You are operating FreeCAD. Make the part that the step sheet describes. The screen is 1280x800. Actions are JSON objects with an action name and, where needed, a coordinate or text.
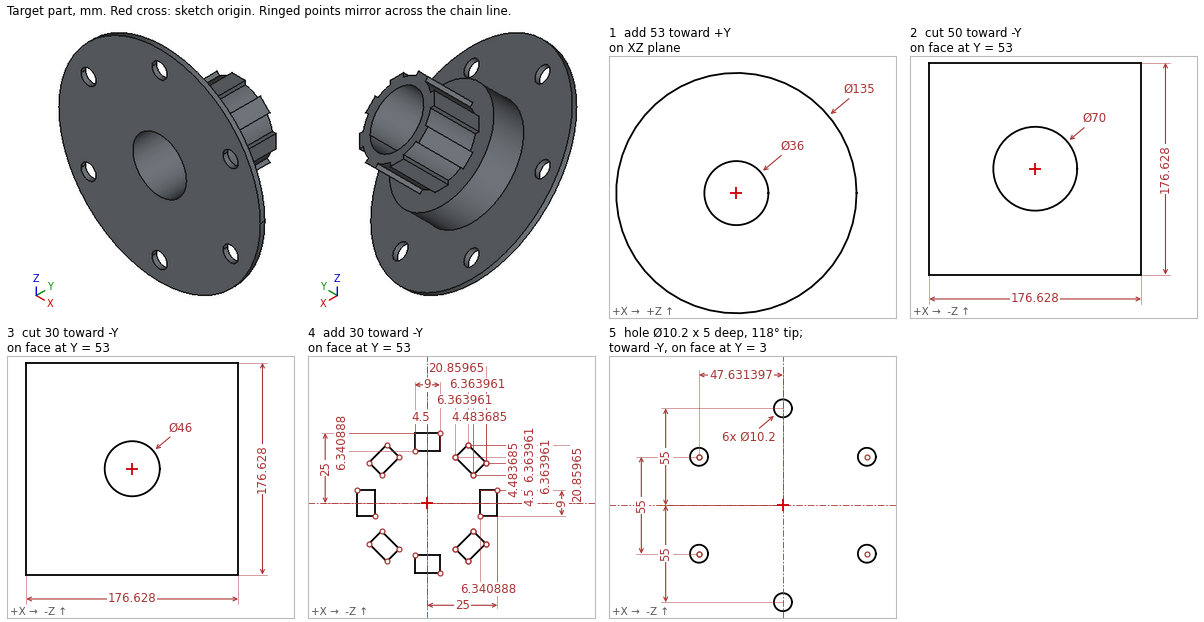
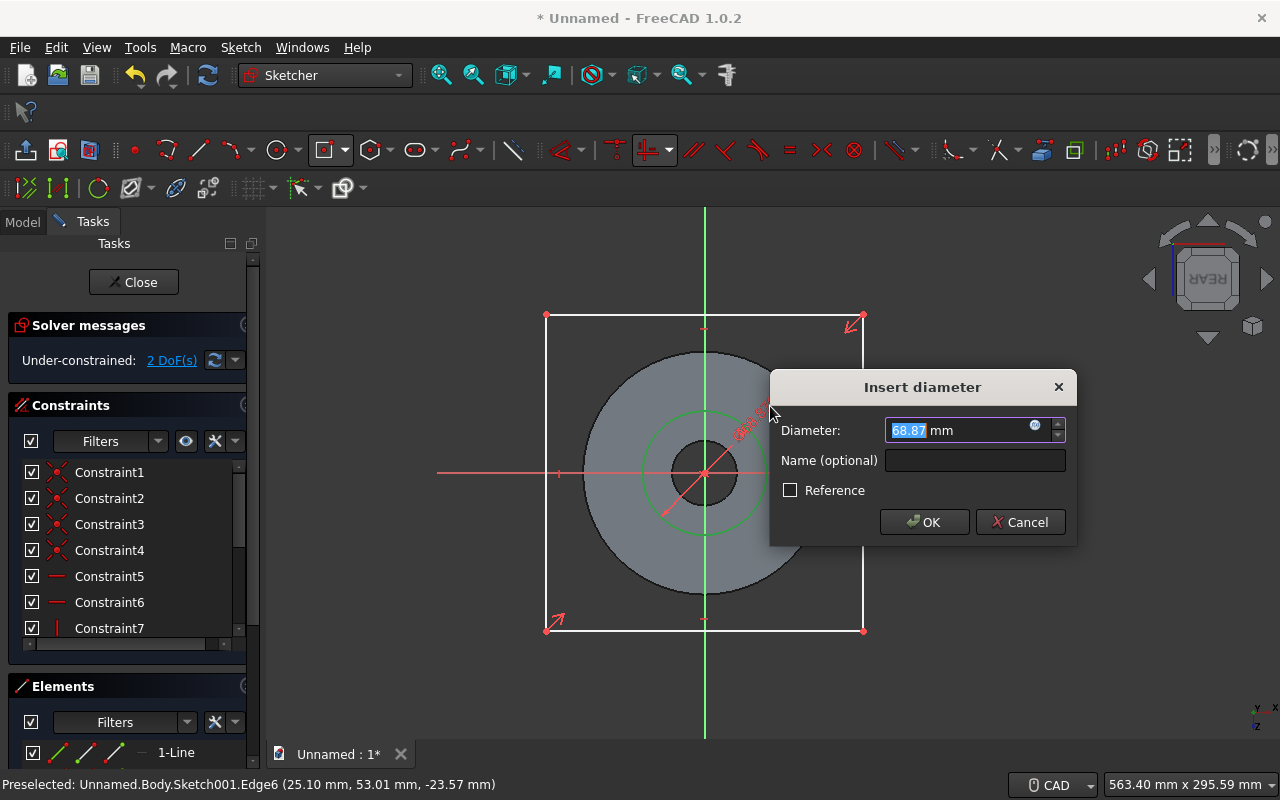
{"action": "type", "text": "70"}
{"action": "key", "text": "Return"}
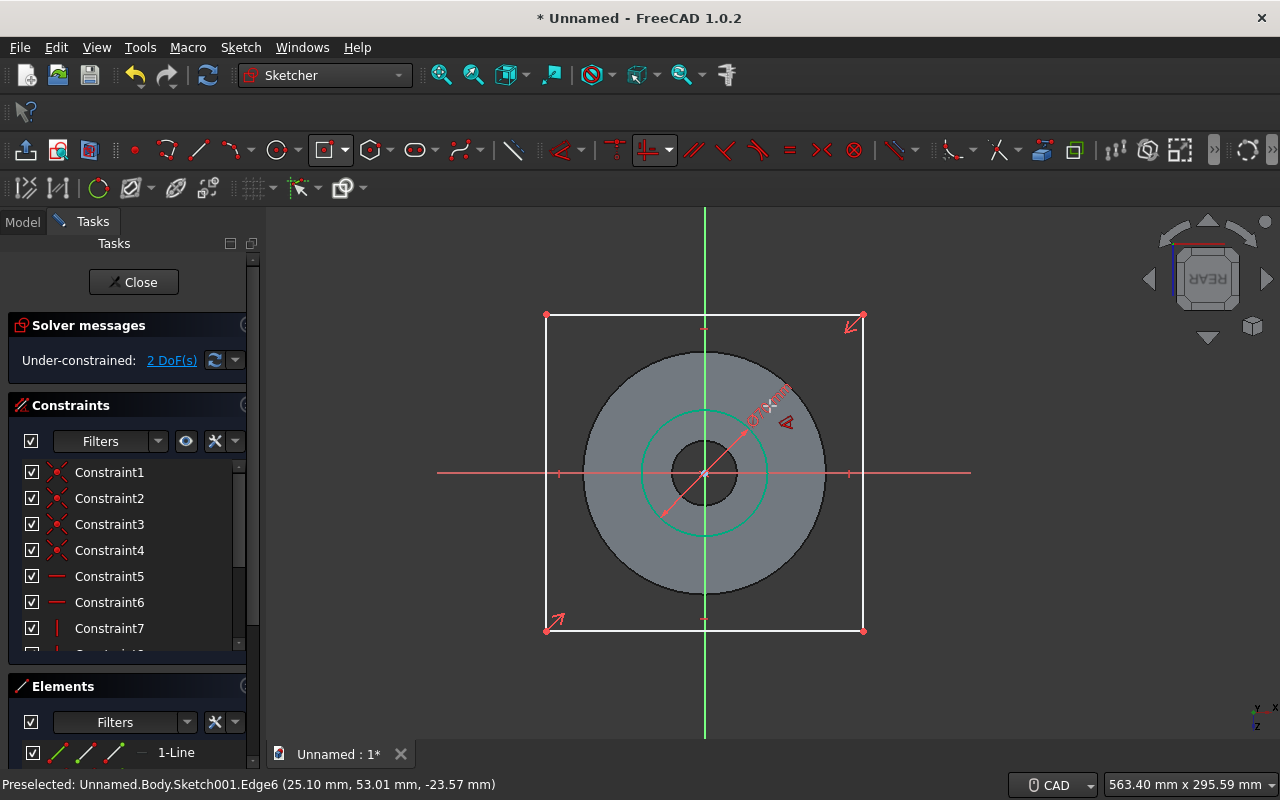
{"action": "left_click", "coordinate": [641, 631]}
{"action": "left_click", "coordinate": [632, 665]}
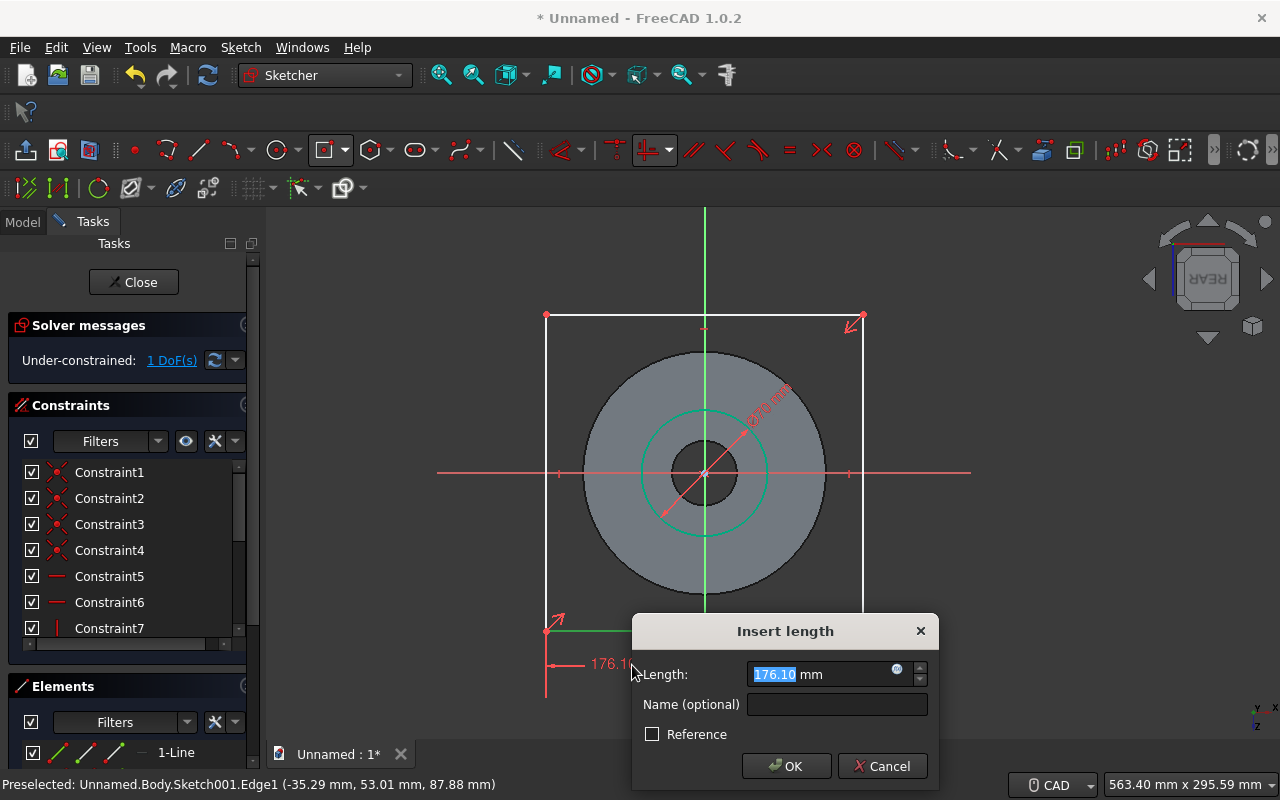
{"action": "type", "text": "176.628"}
{"action": "key", "text": "Return"}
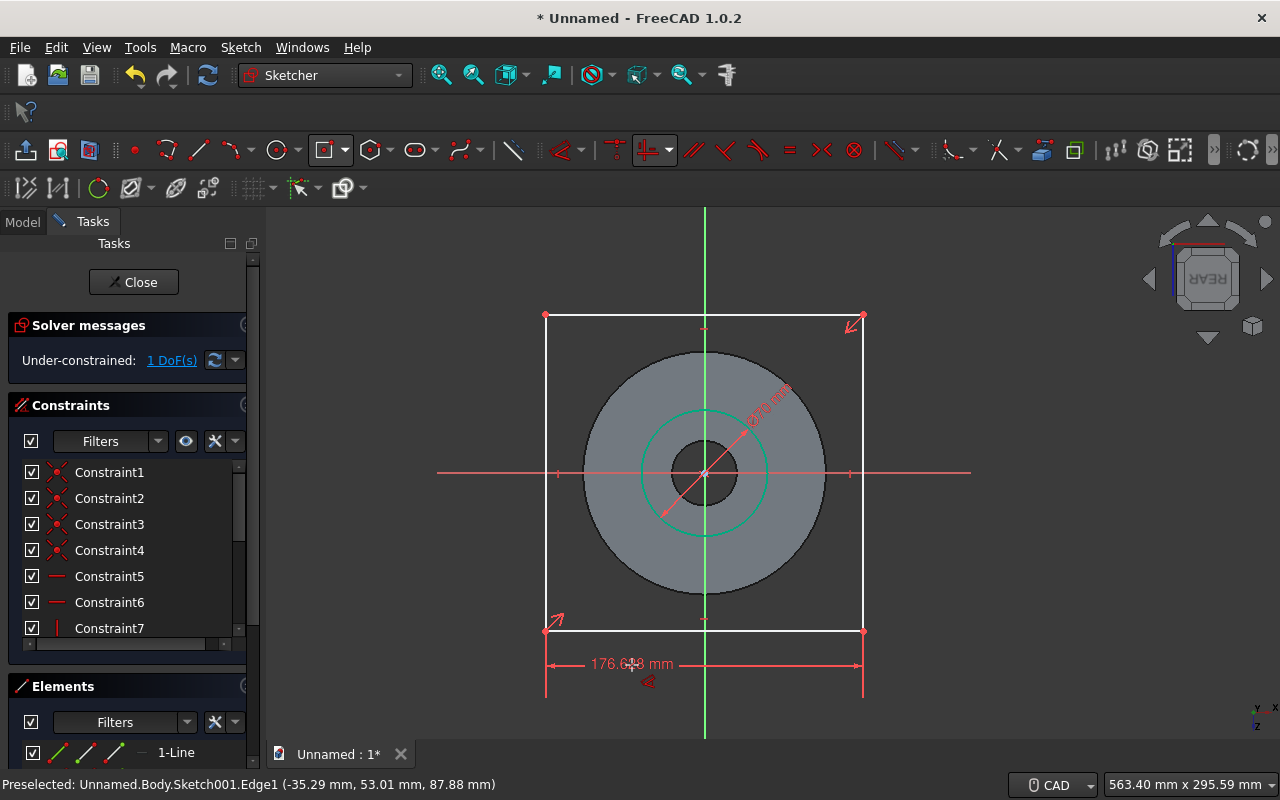
{"action": "left_click", "coordinate": [863, 536]}
{"action": "left_click", "coordinate": [897, 400]}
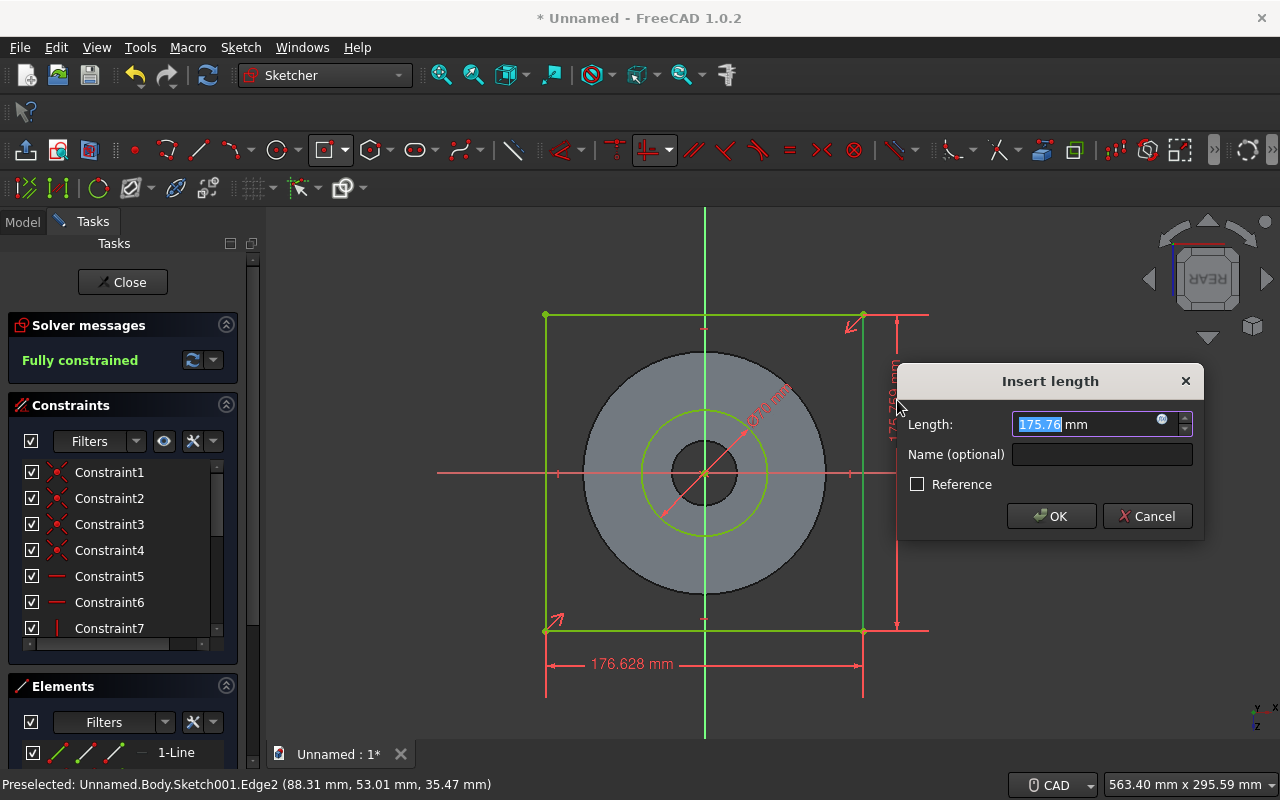
{"action": "type", "text": "176.628"}
{"action": "key", "text": "Return"}
{"action": "key", "text": "Escape"}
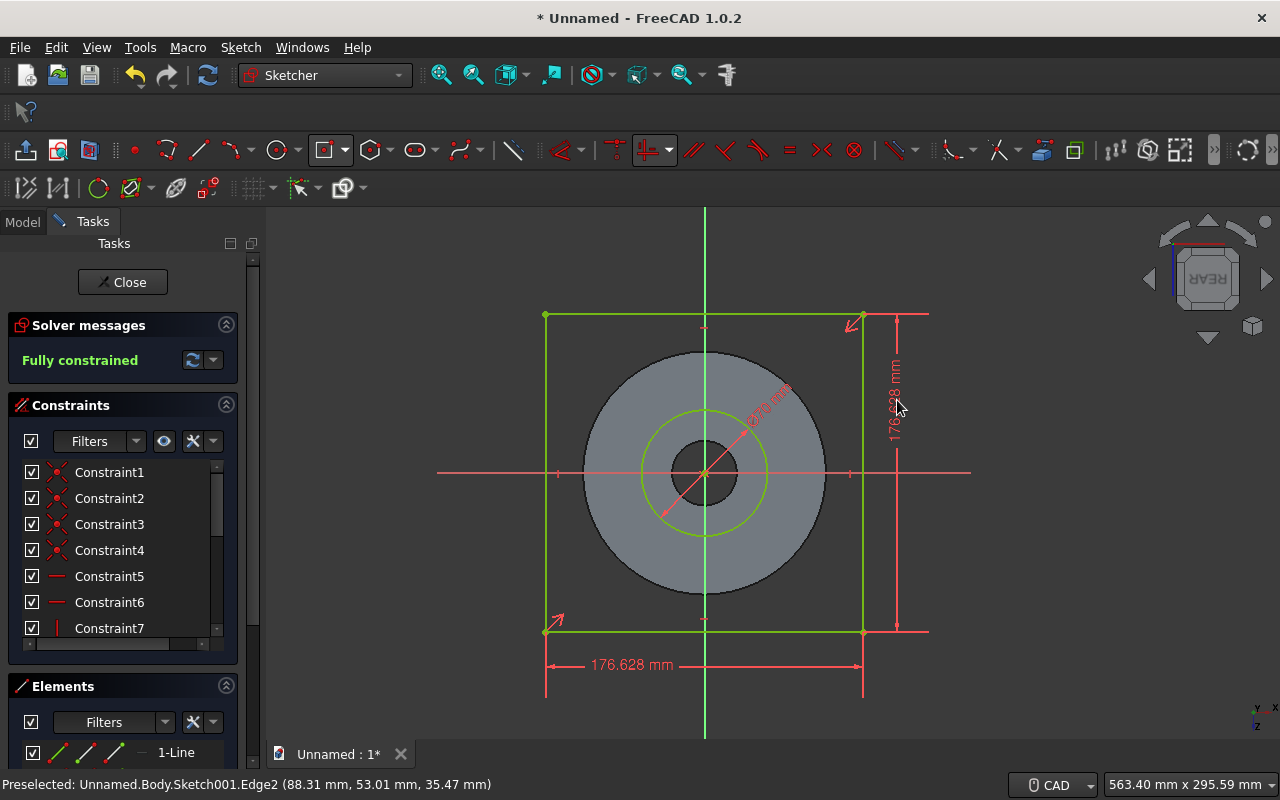
{"action": "left_click", "coordinate": [123, 282]}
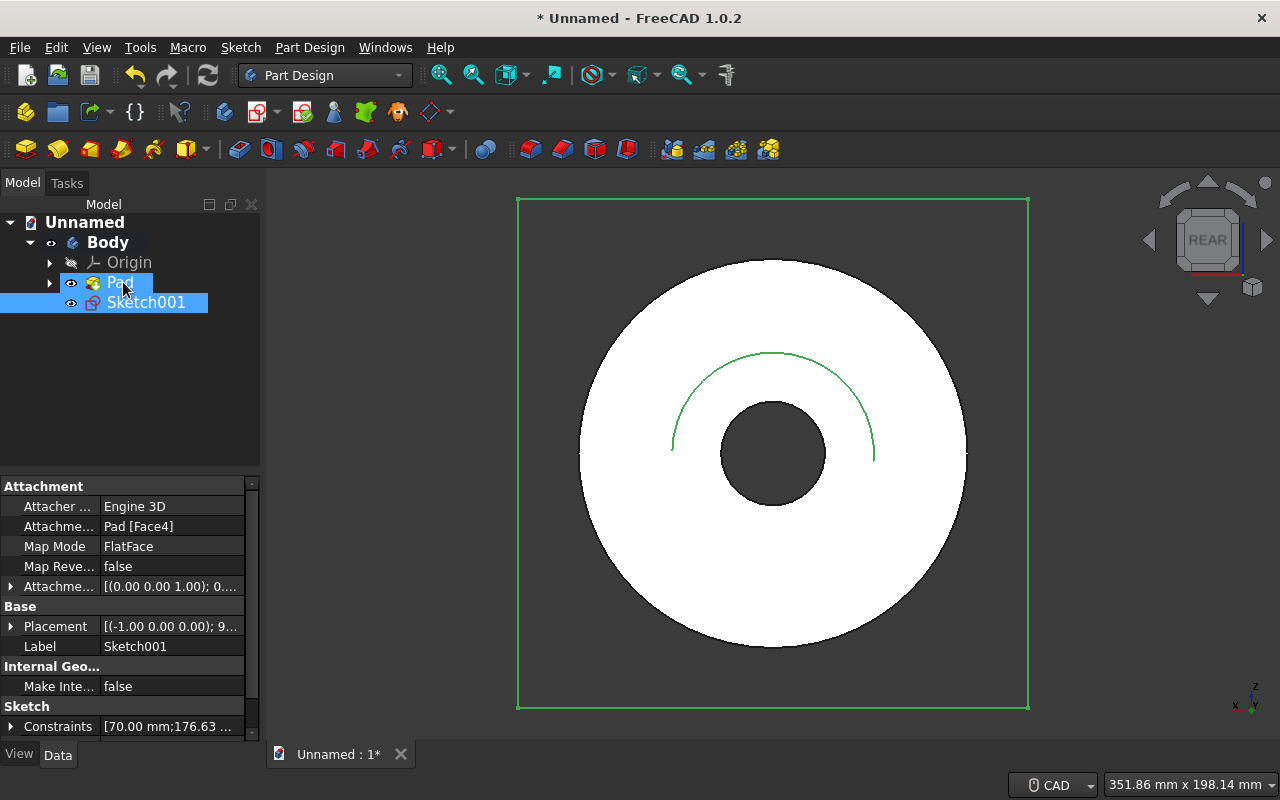
{"action": "left_click", "coordinate": [240, 150]}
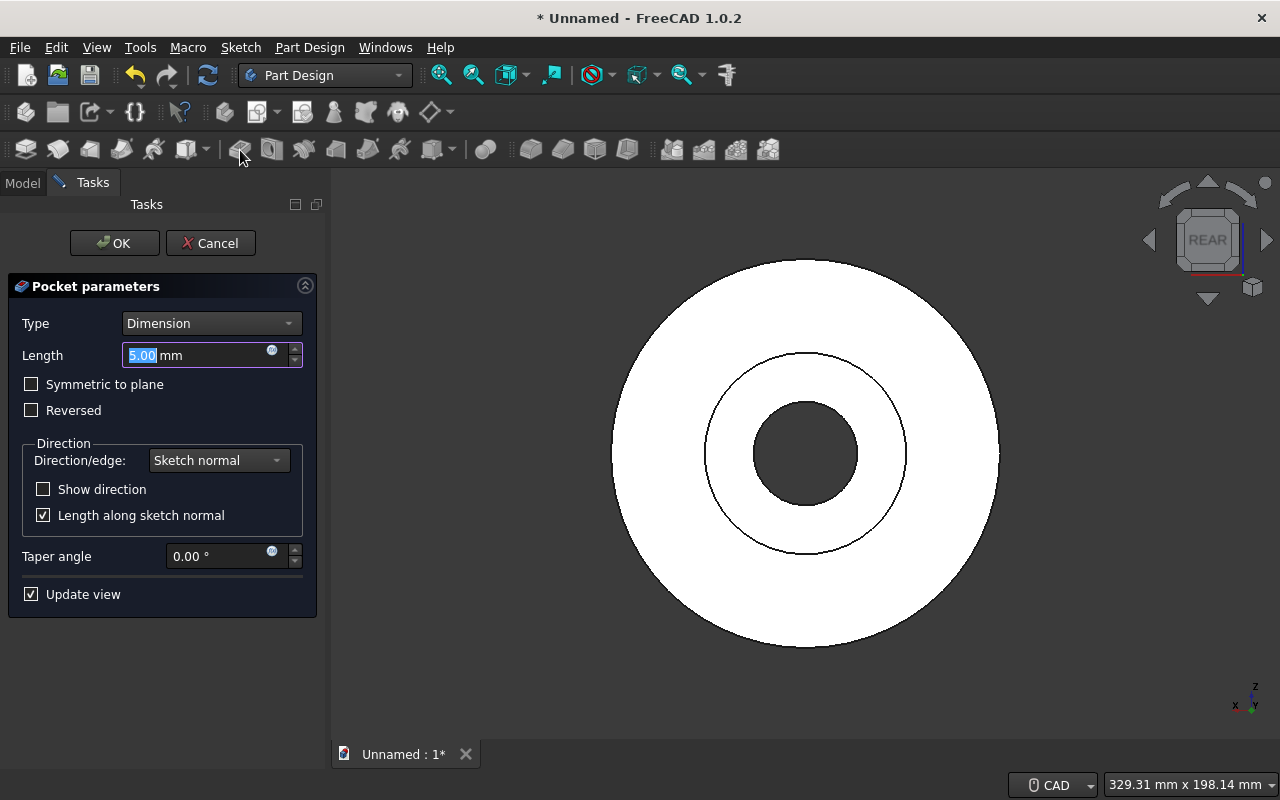
{"action": "type", "text": "50"}
{"action": "key", "text": "Tab"}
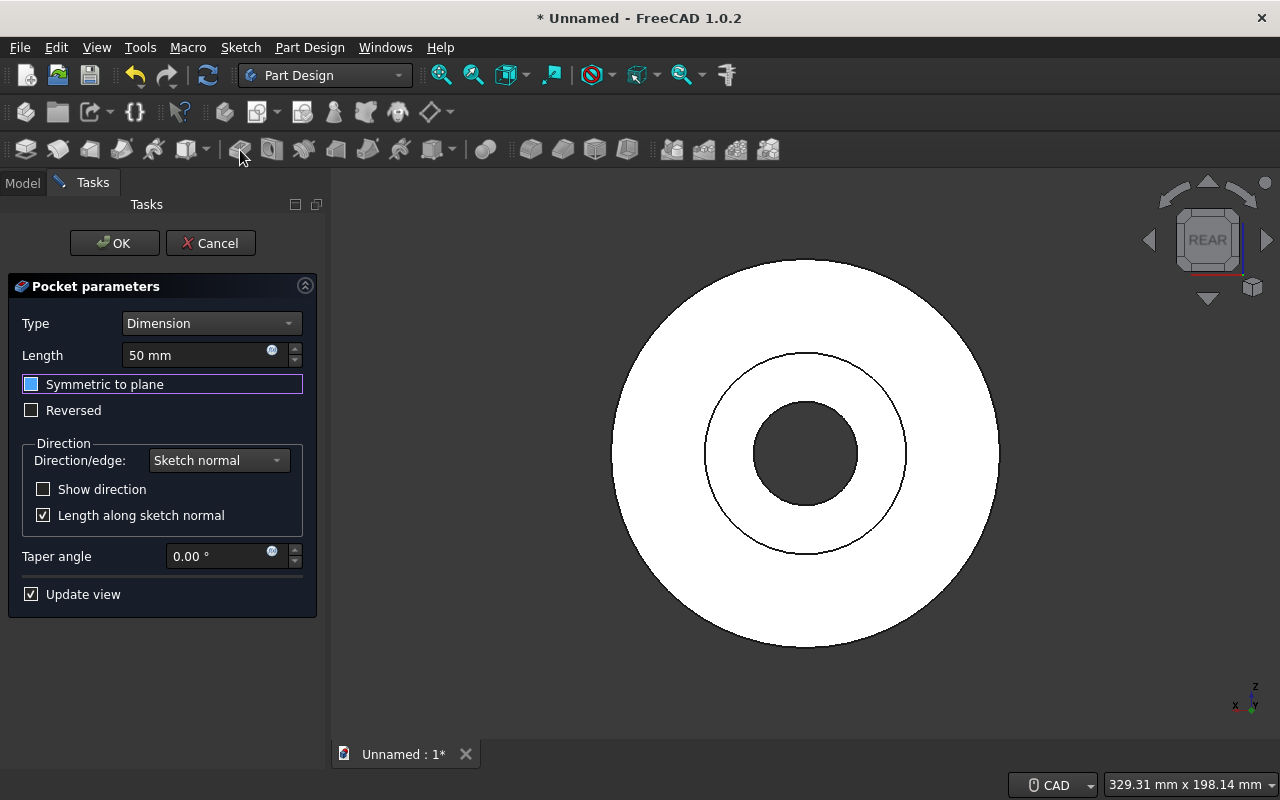
{"action": "left_click", "coordinate": [115, 243]}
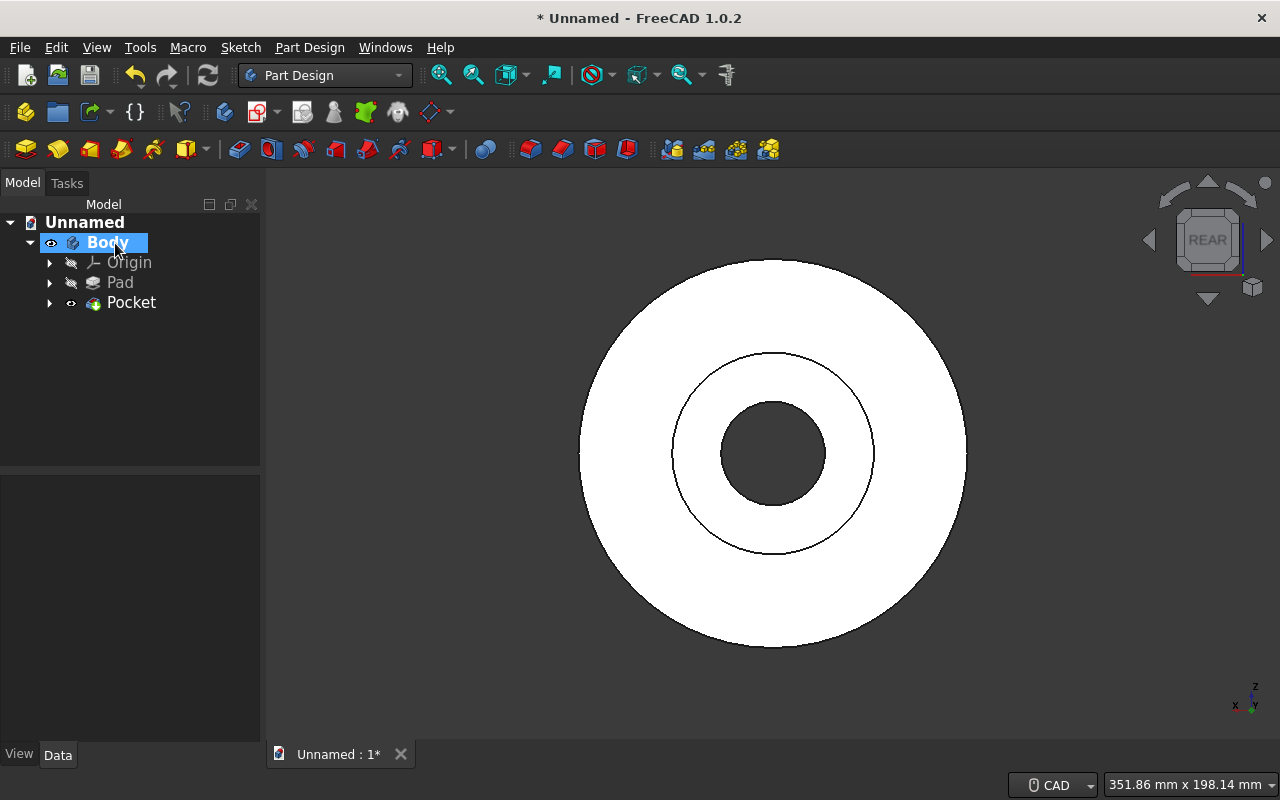
{"action": "left_click", "coordinate": [831, 510]}